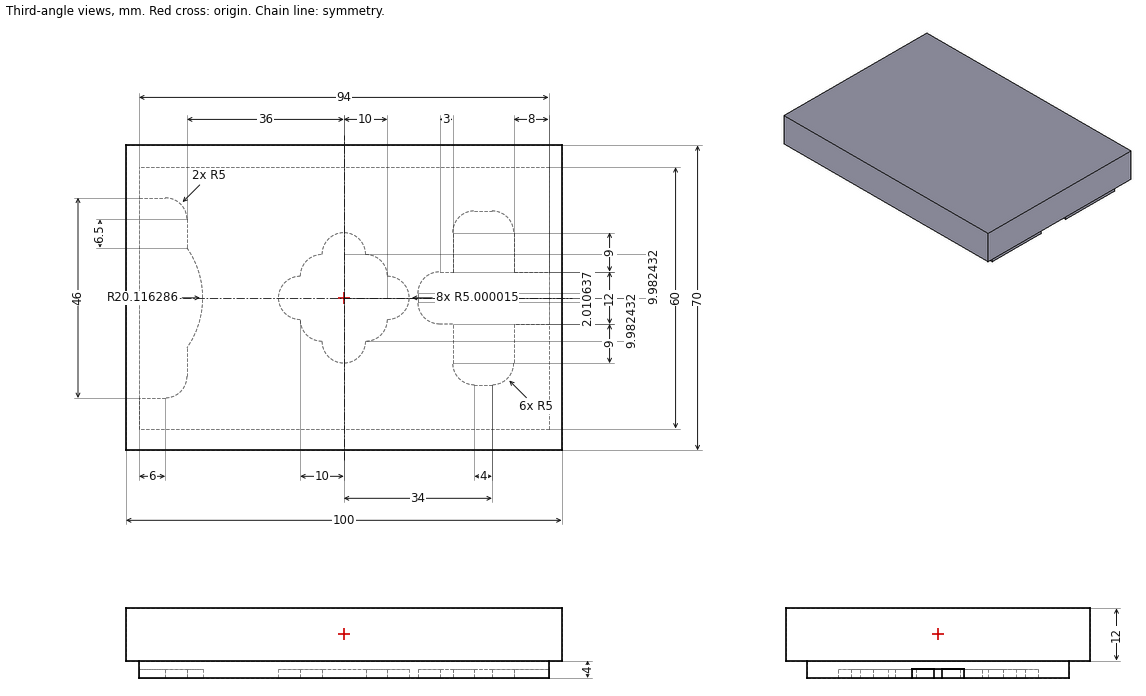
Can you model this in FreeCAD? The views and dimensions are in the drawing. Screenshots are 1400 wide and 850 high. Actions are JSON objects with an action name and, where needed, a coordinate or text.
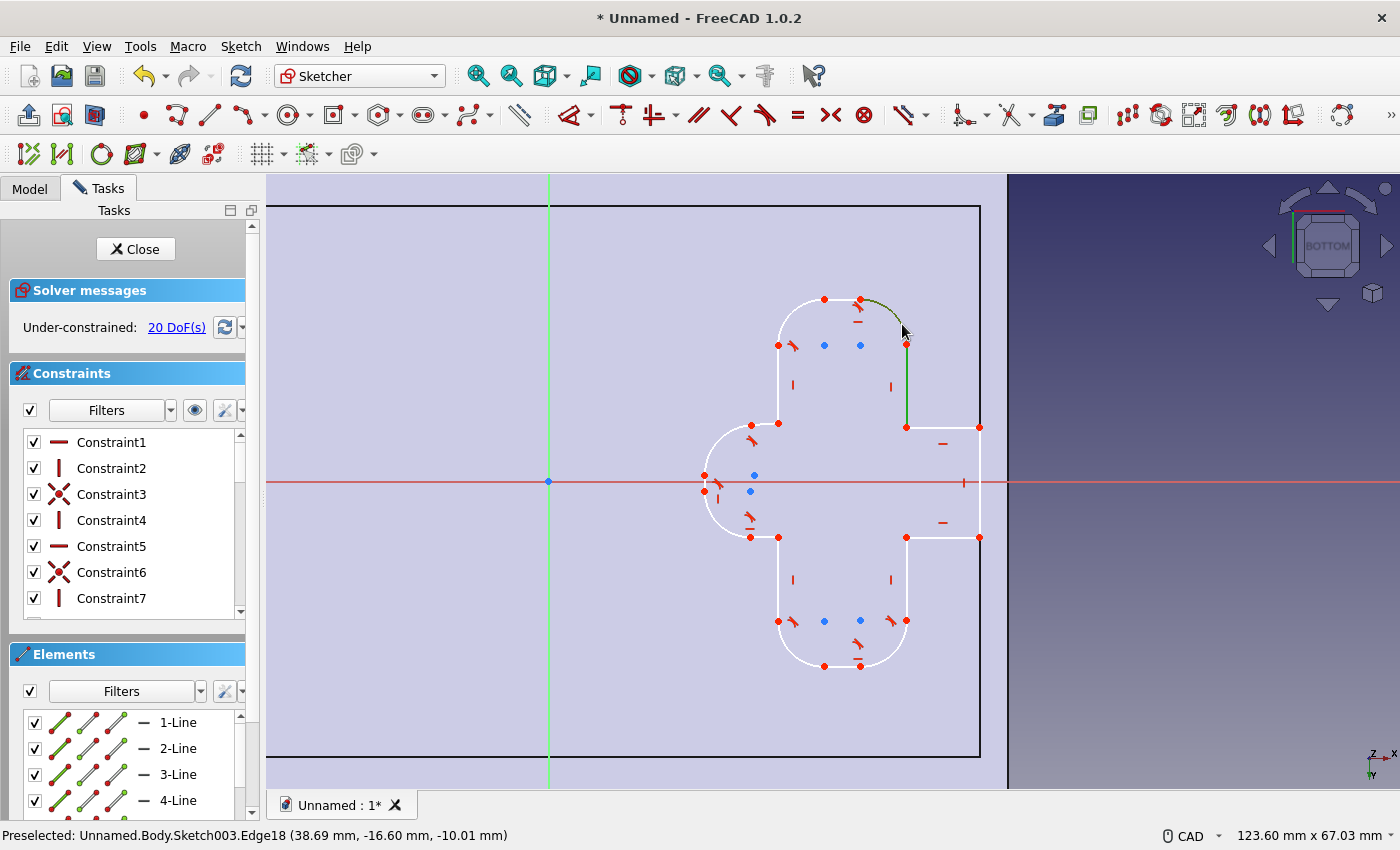
{"action": "left_click", "coordinate": [765, 116]}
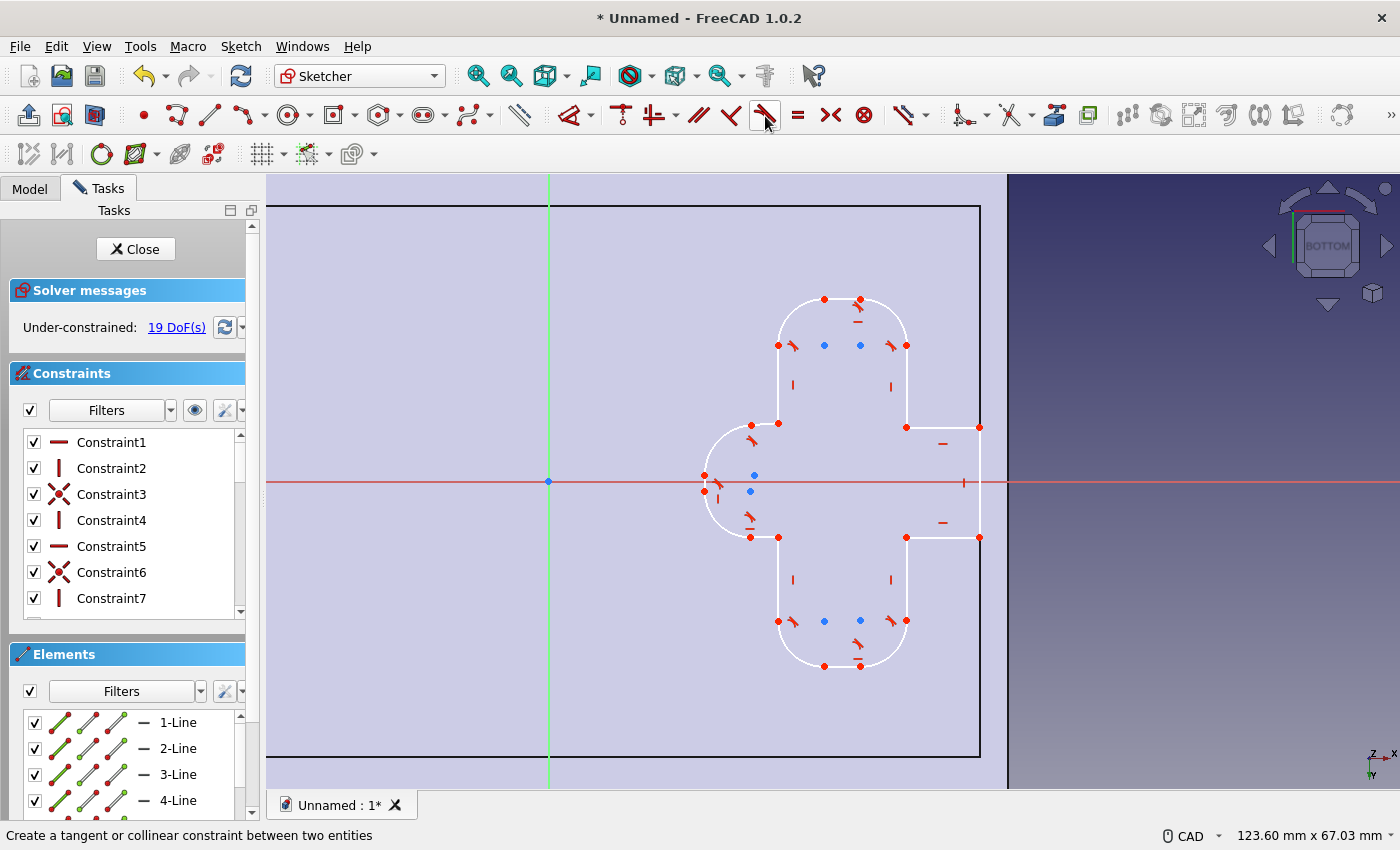
{"action": "left_click", "coordinate": [803, 304]}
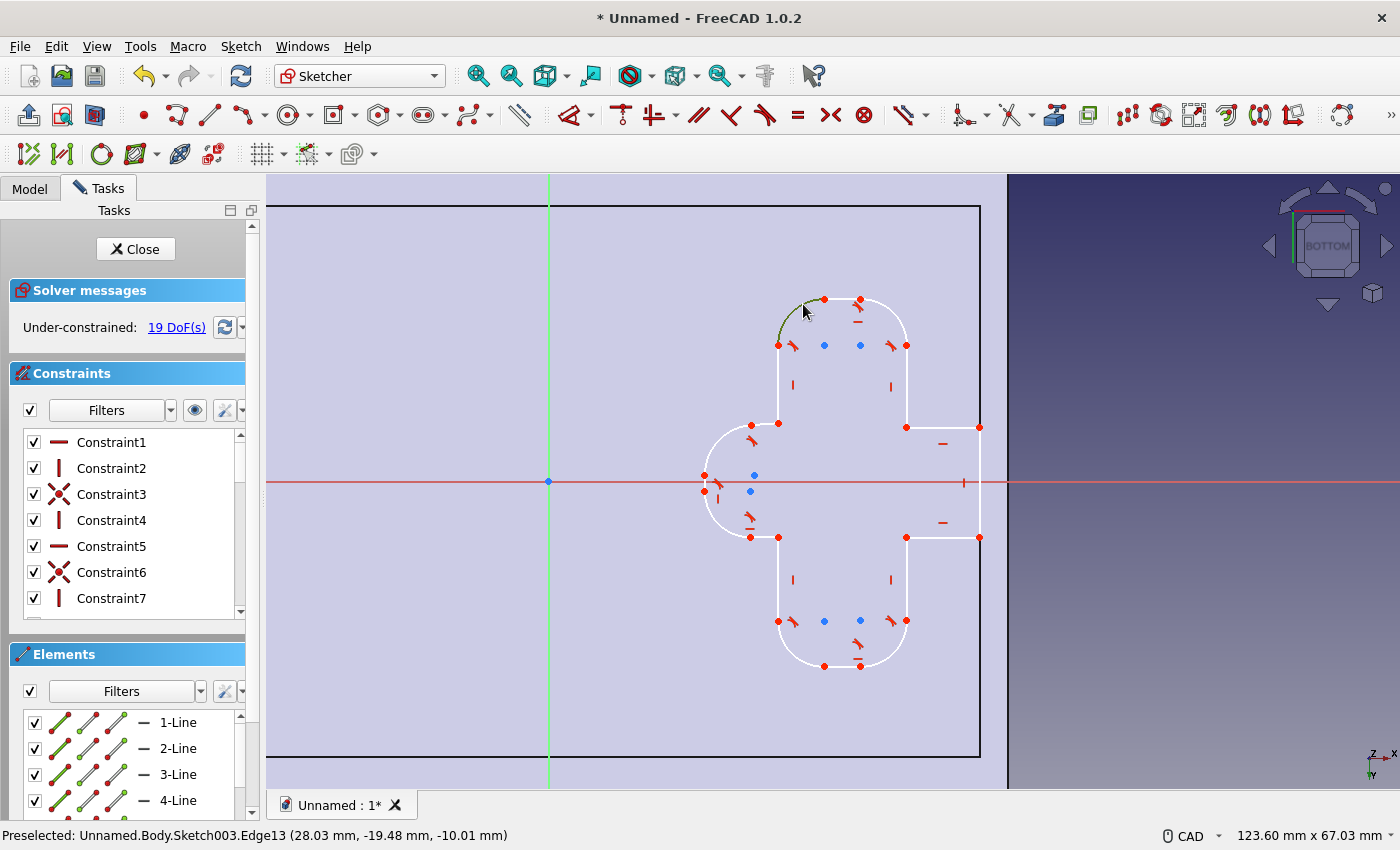
{"action": "left_click", "coordinate": [730, 432]}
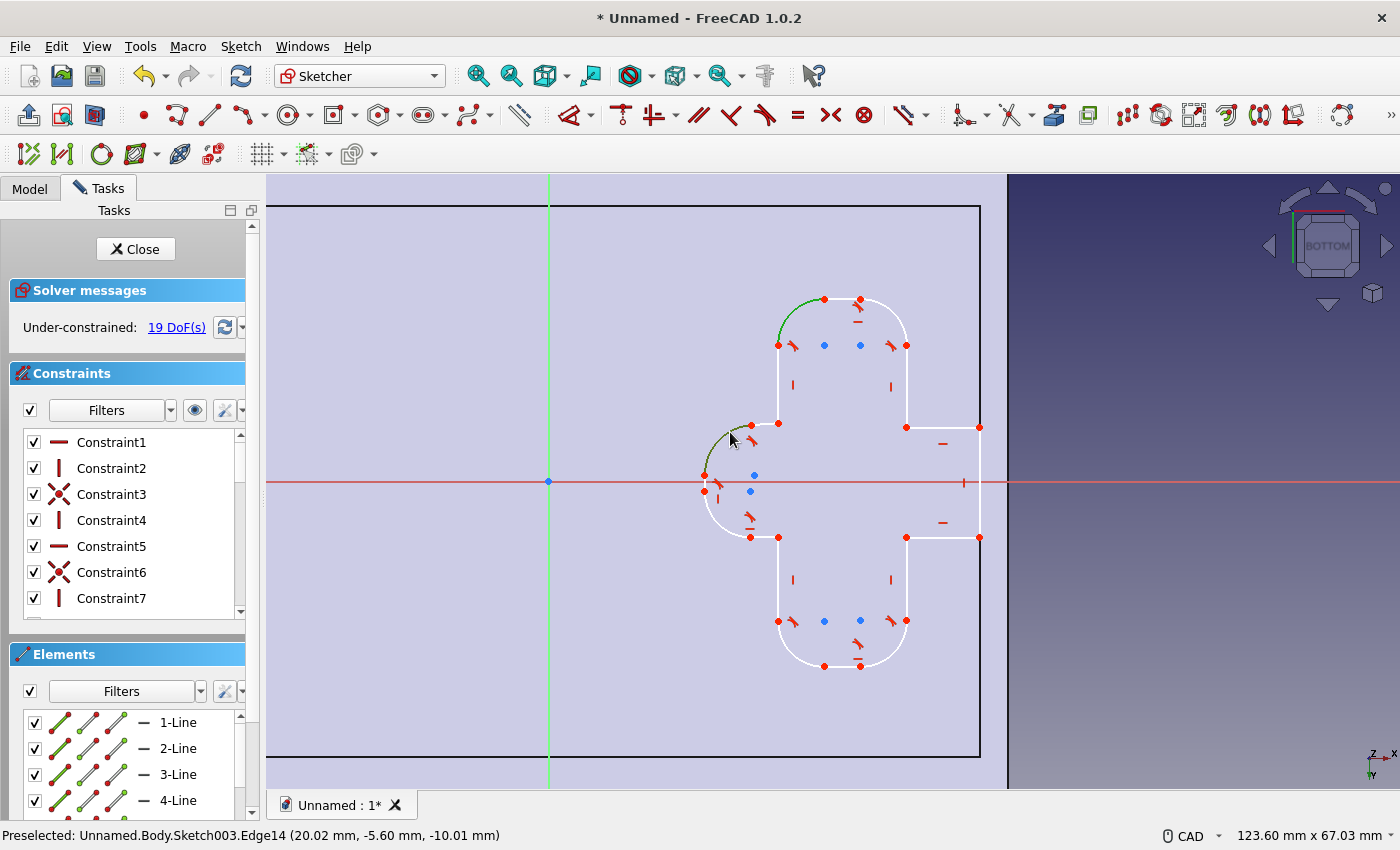
{"action": "left_click", "coordinate": [710, 512]}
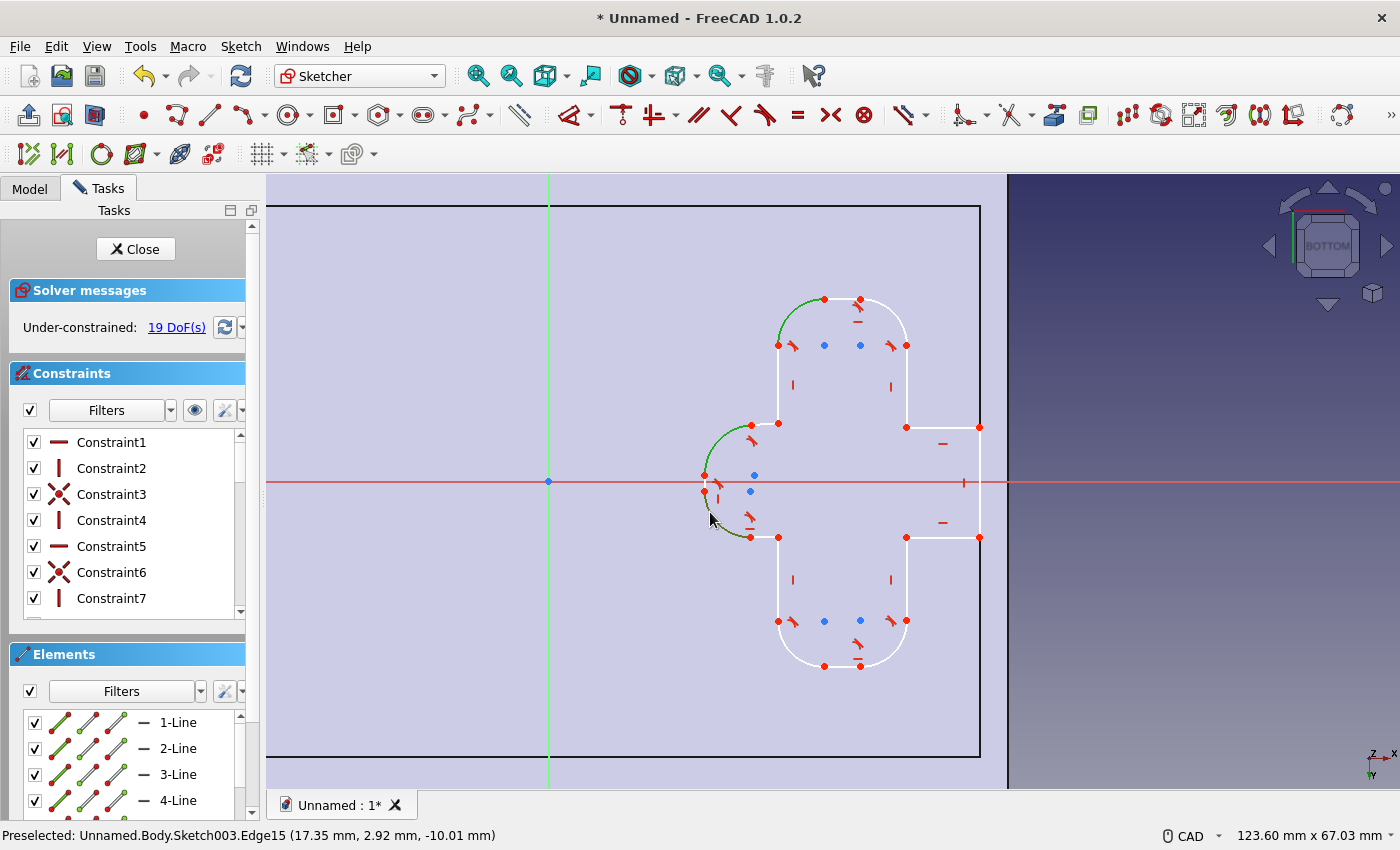
{"action": "left_click", "coordinate": [783, 642]}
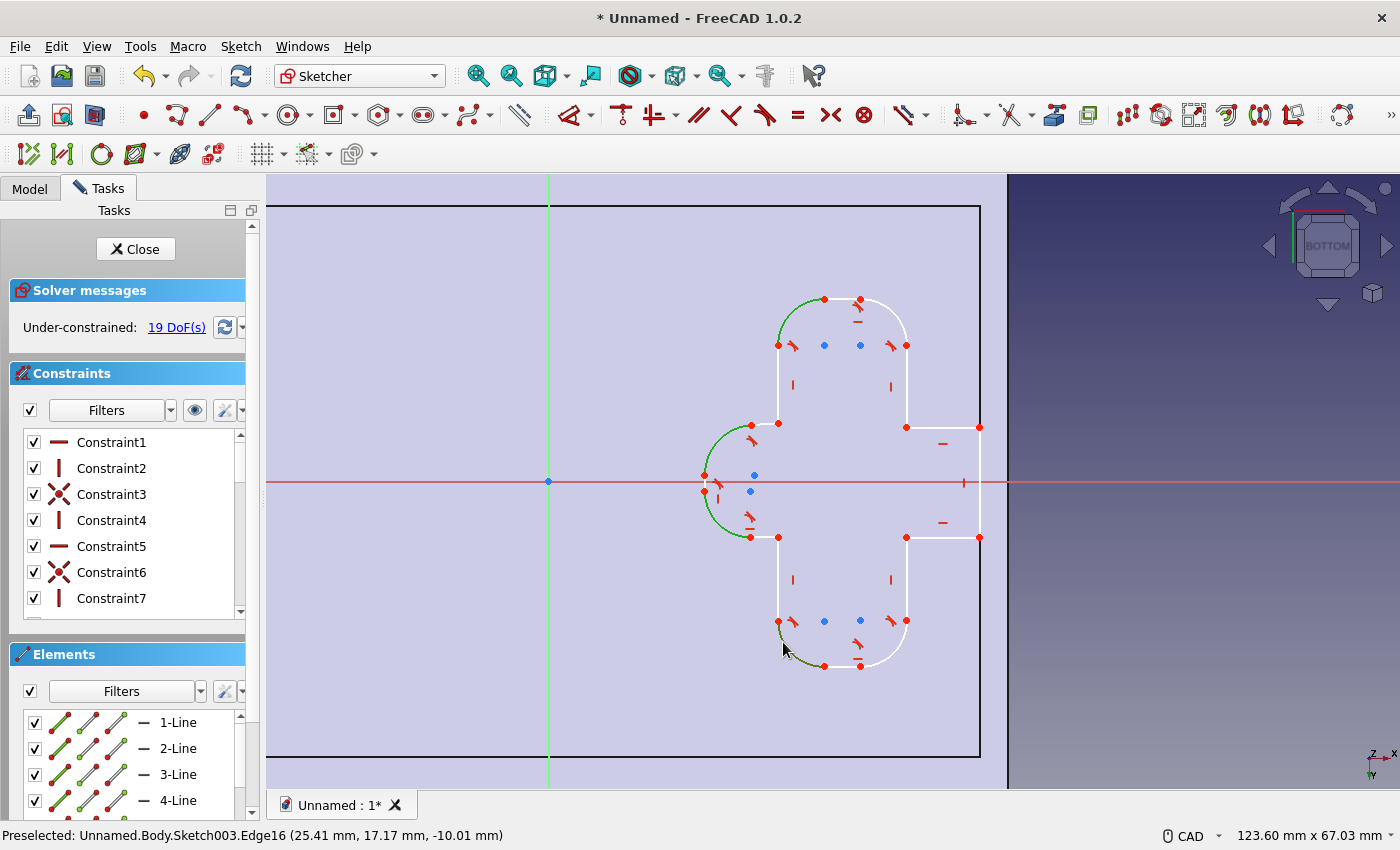
{"action": "left_click", "coordinate": [882, 662]}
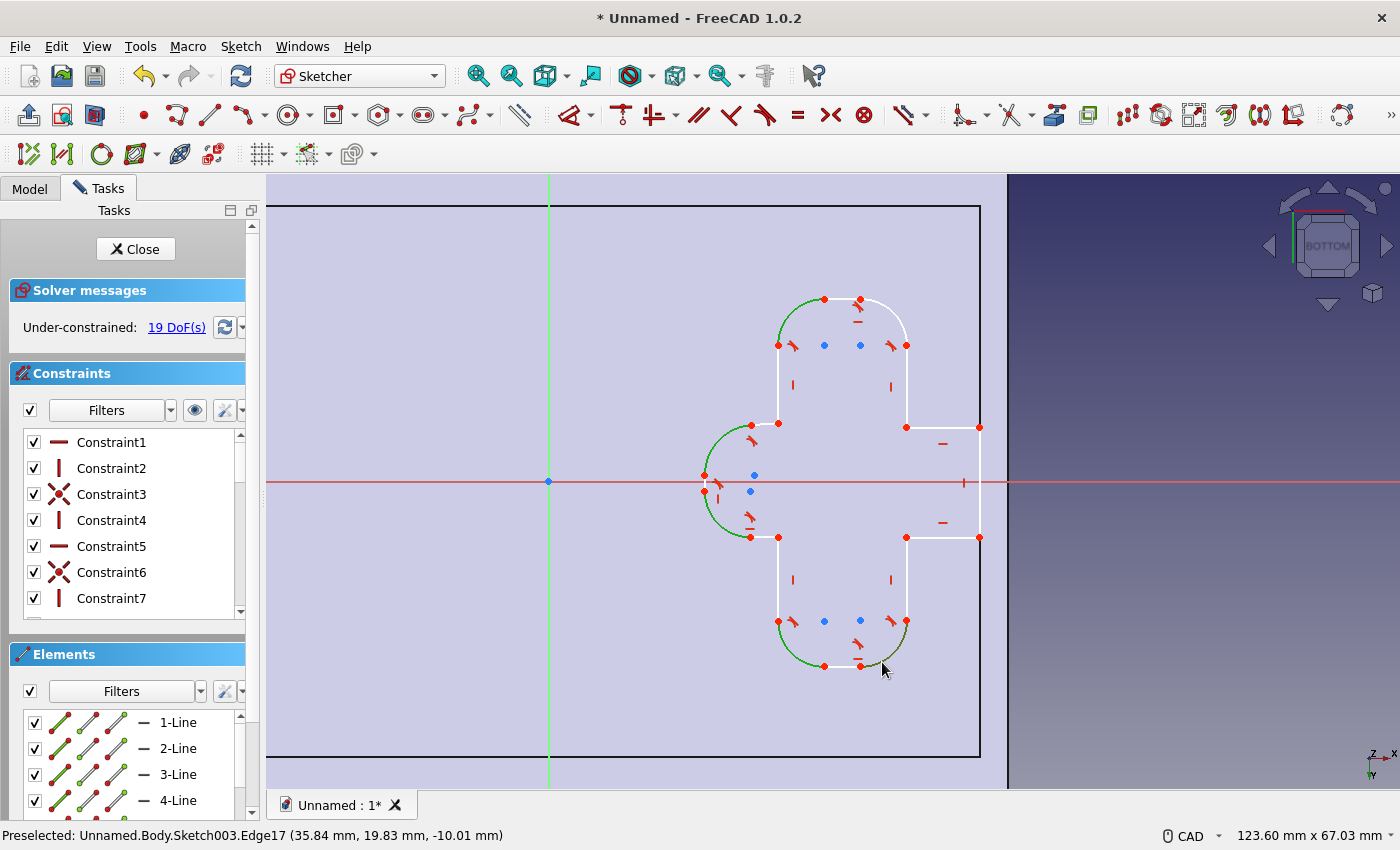
{"action": "left_click", "coordinate": [902, 324]}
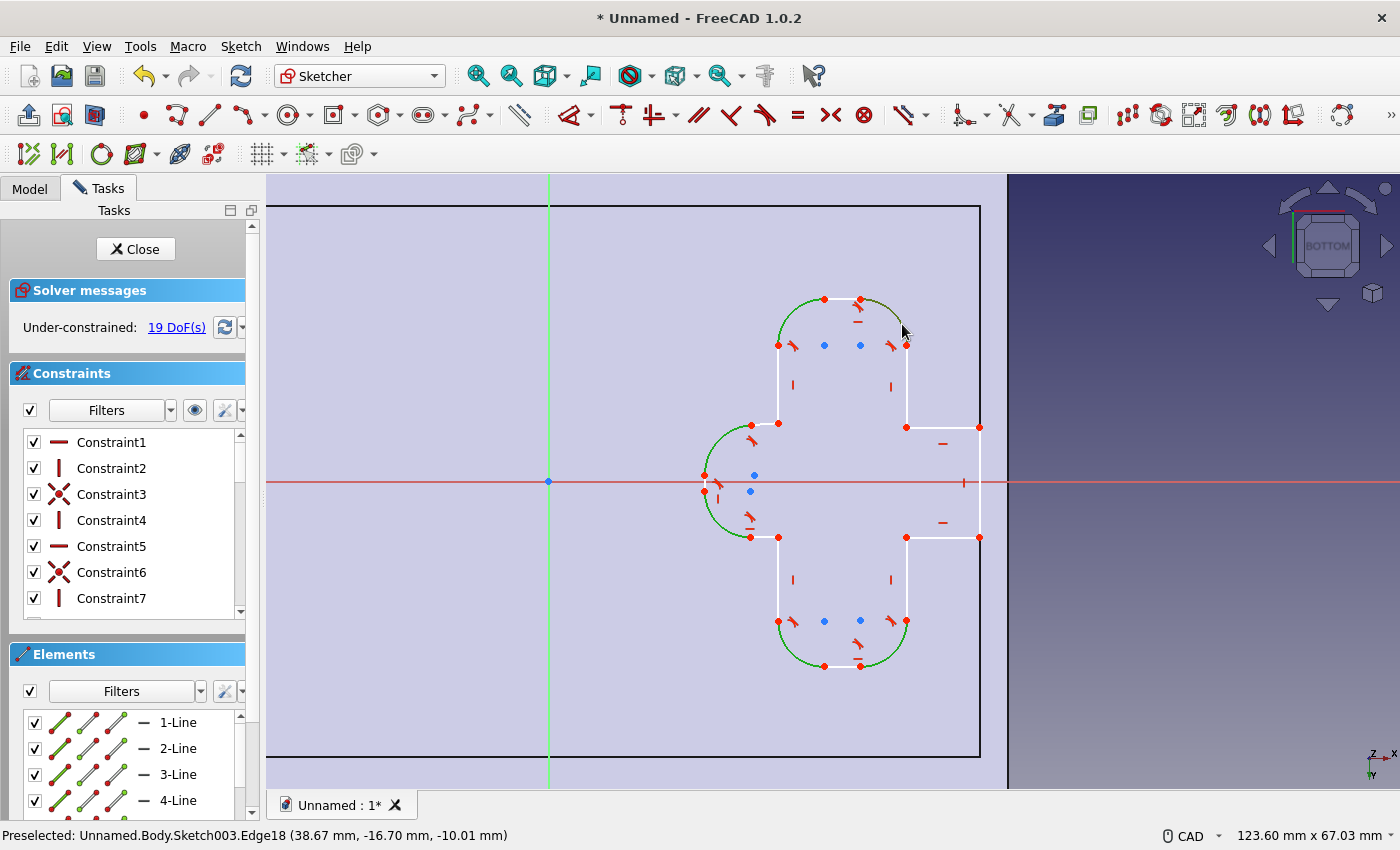
{"action": "left_click", "coordinate": [798, 116]}